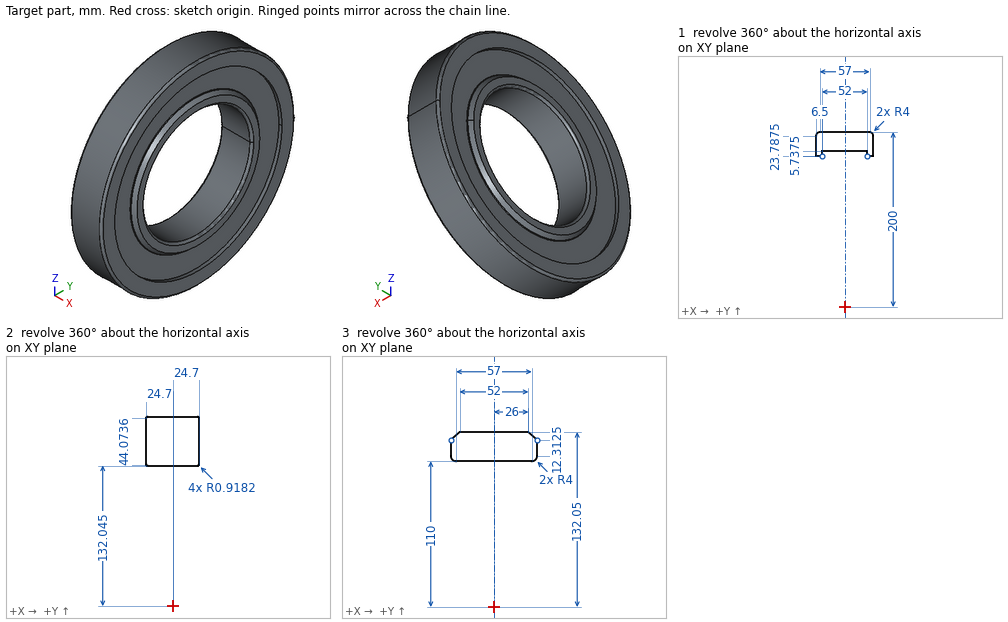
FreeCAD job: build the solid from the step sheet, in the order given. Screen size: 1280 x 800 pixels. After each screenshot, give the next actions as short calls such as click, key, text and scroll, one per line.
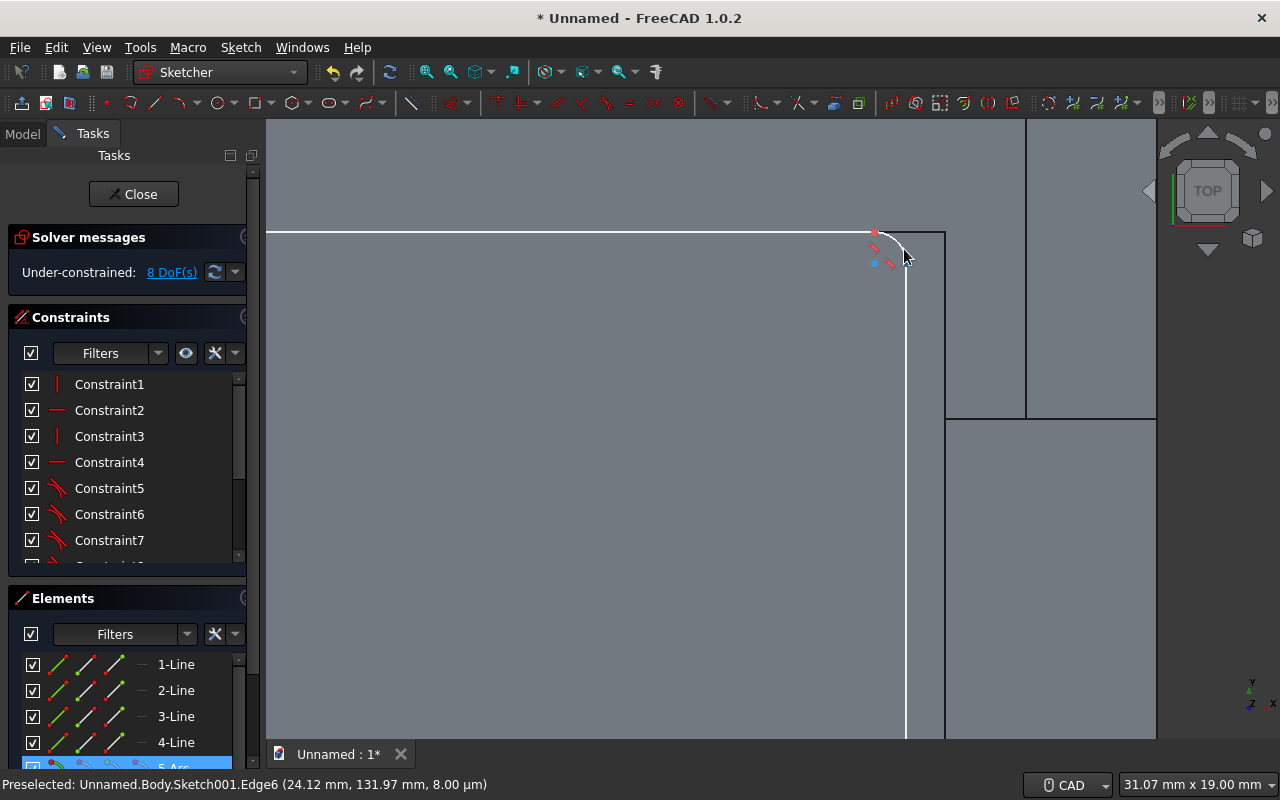
click(903, 249)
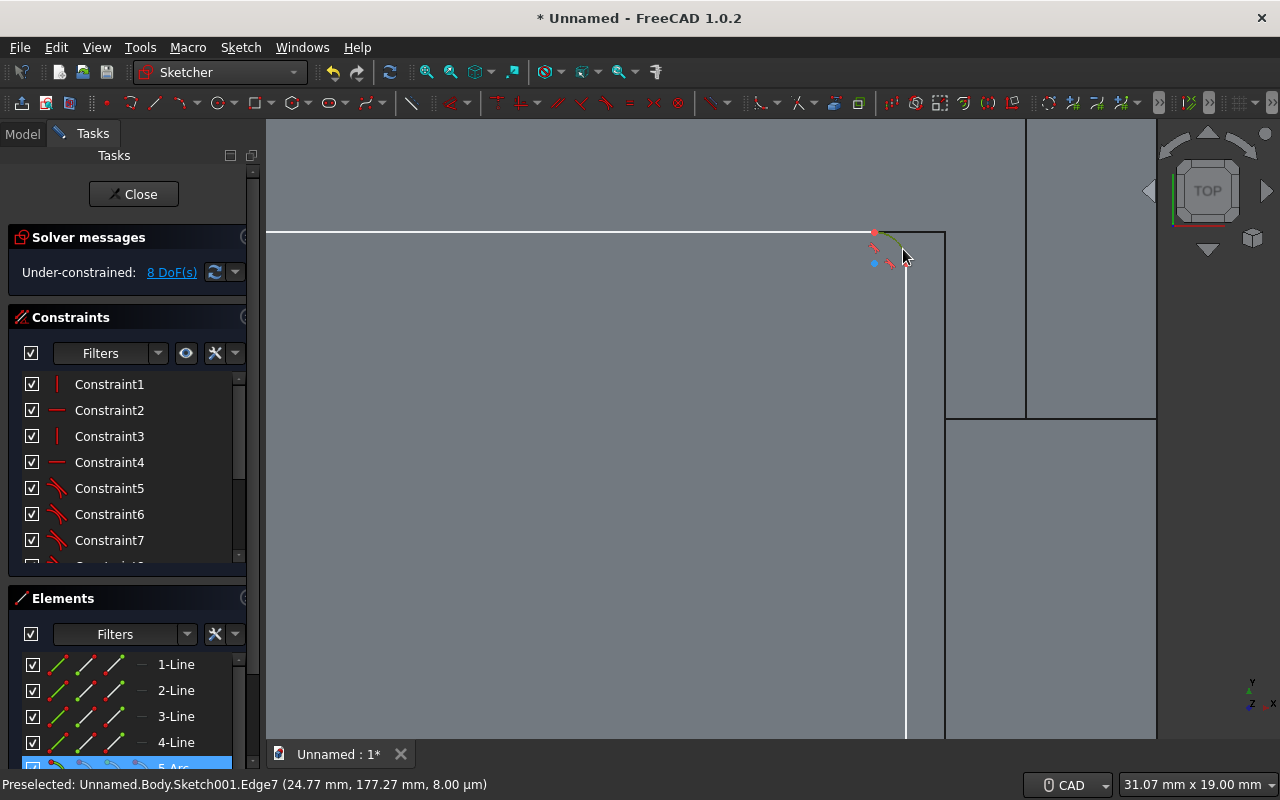
scroll(904, 248, down, 7)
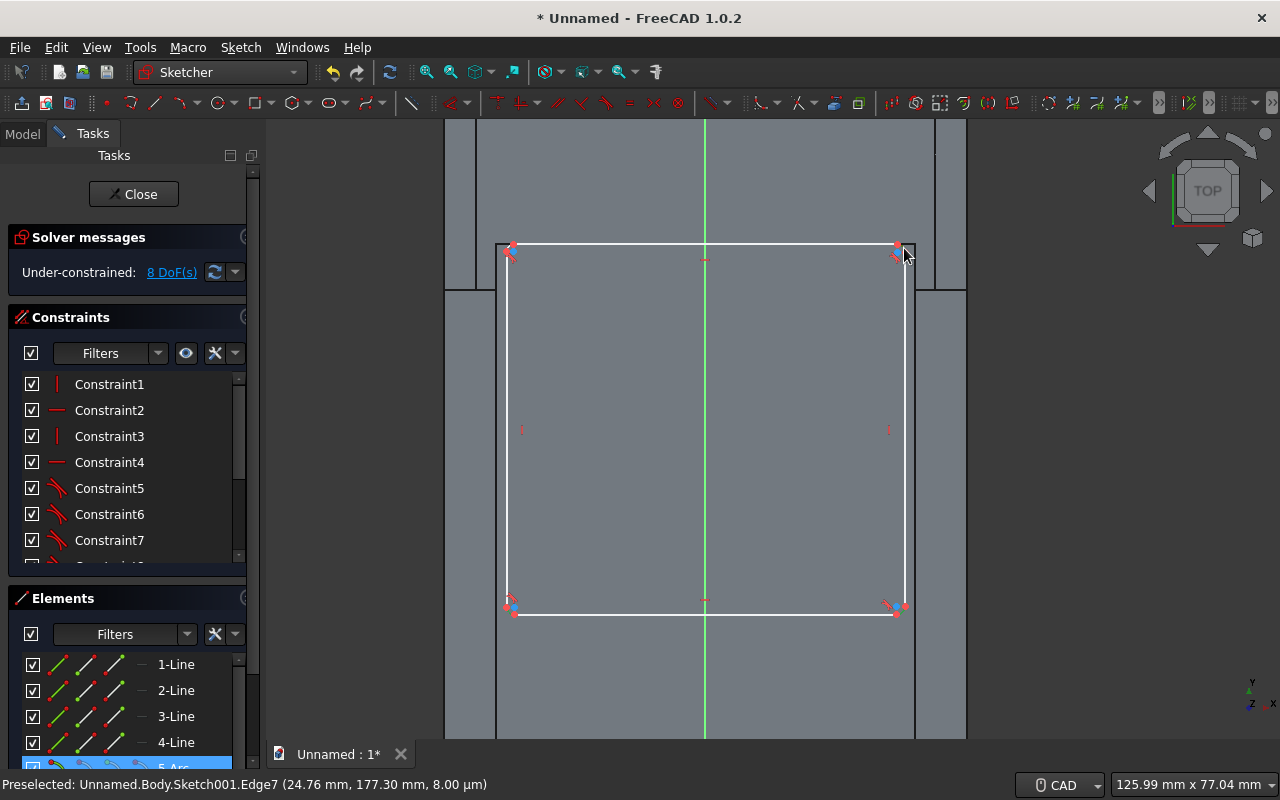
scroll(510, 245, up, 8)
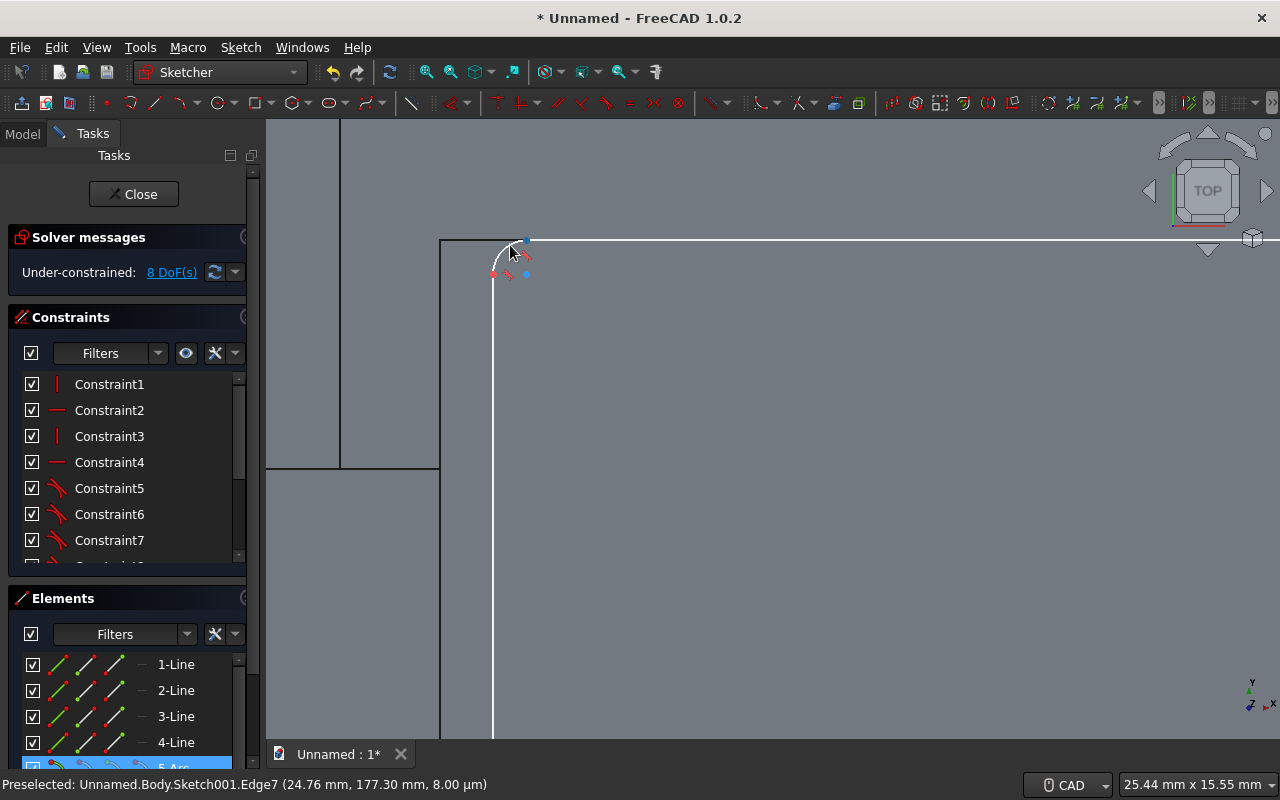
click(511, 244)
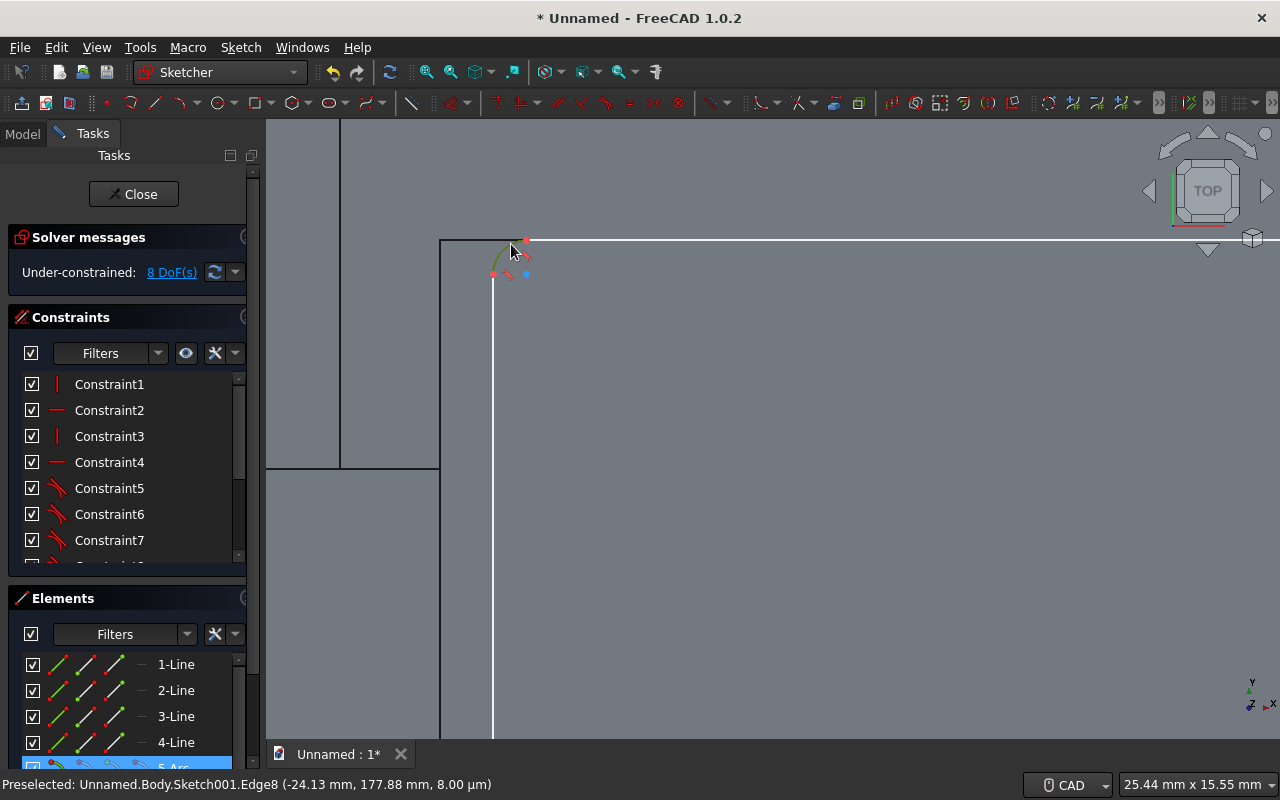
click(630, 104)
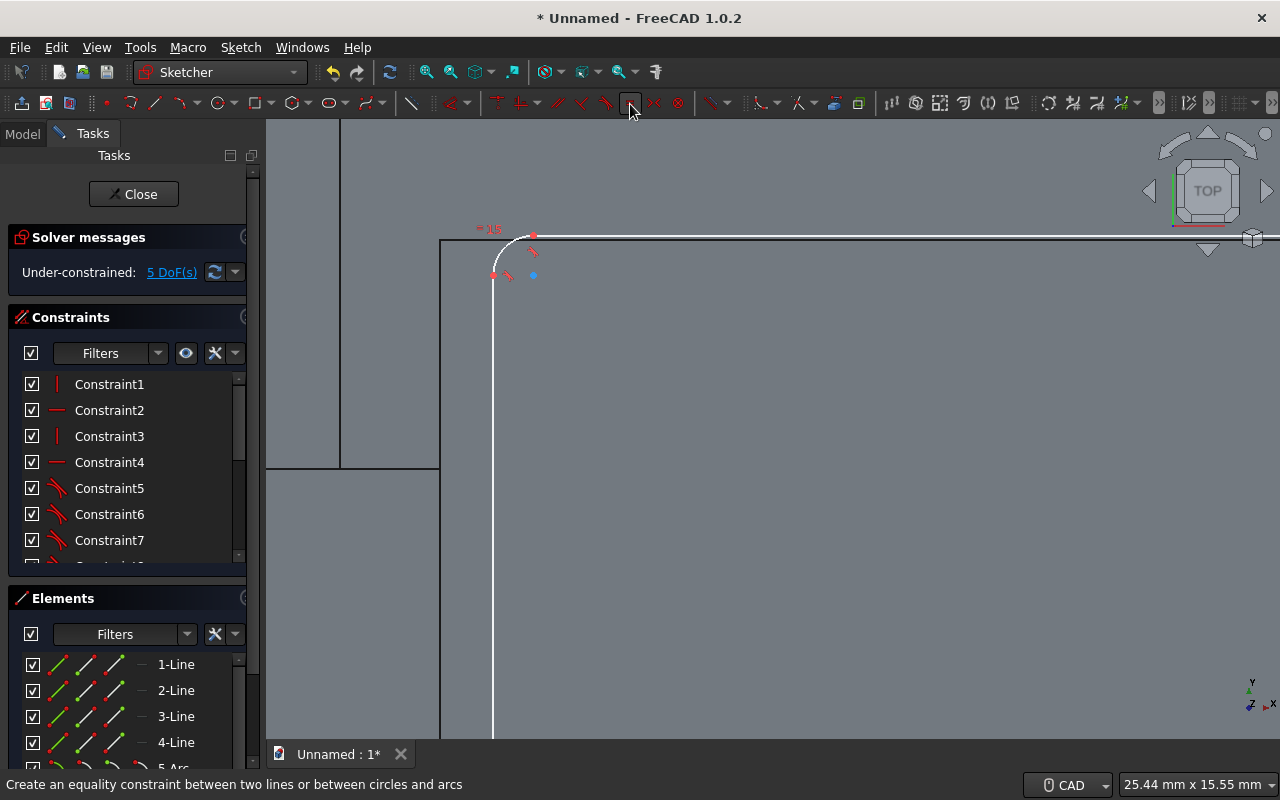
click(450, 104)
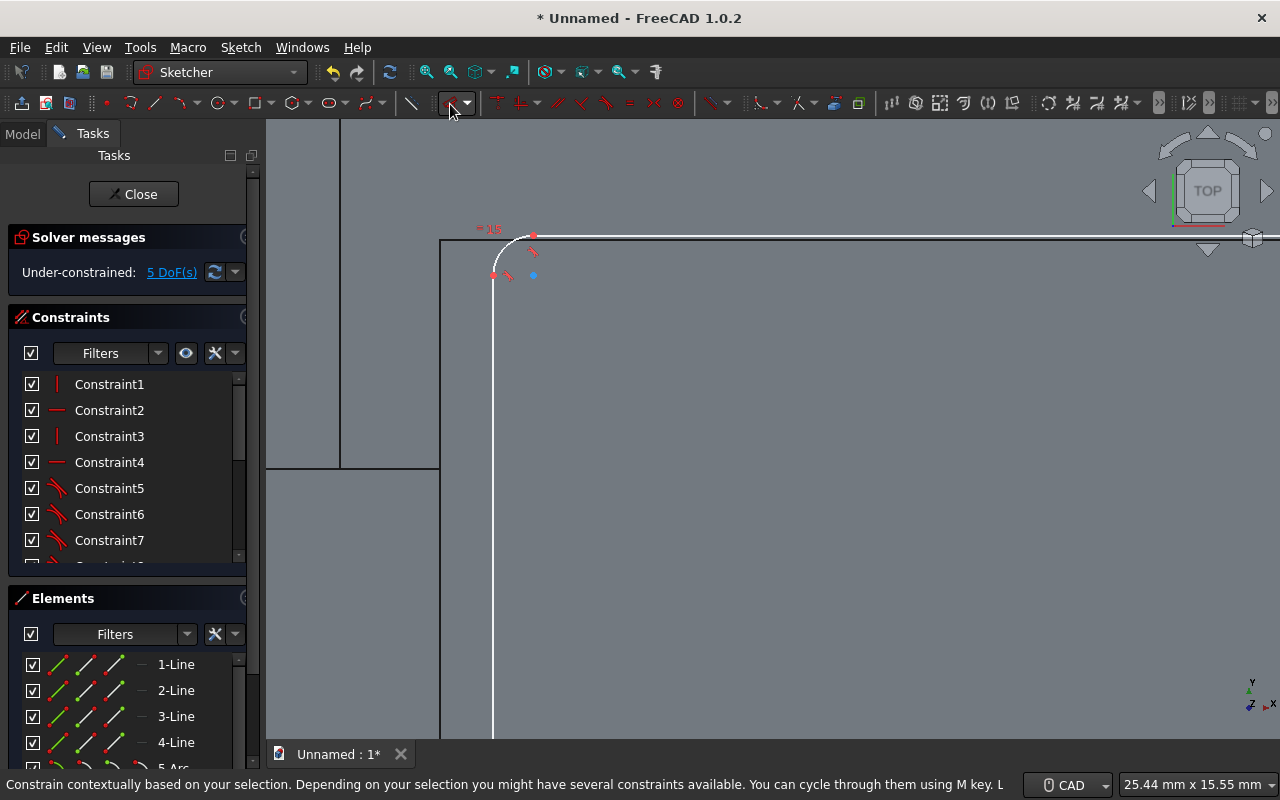
scroll(509, 245, down, 8)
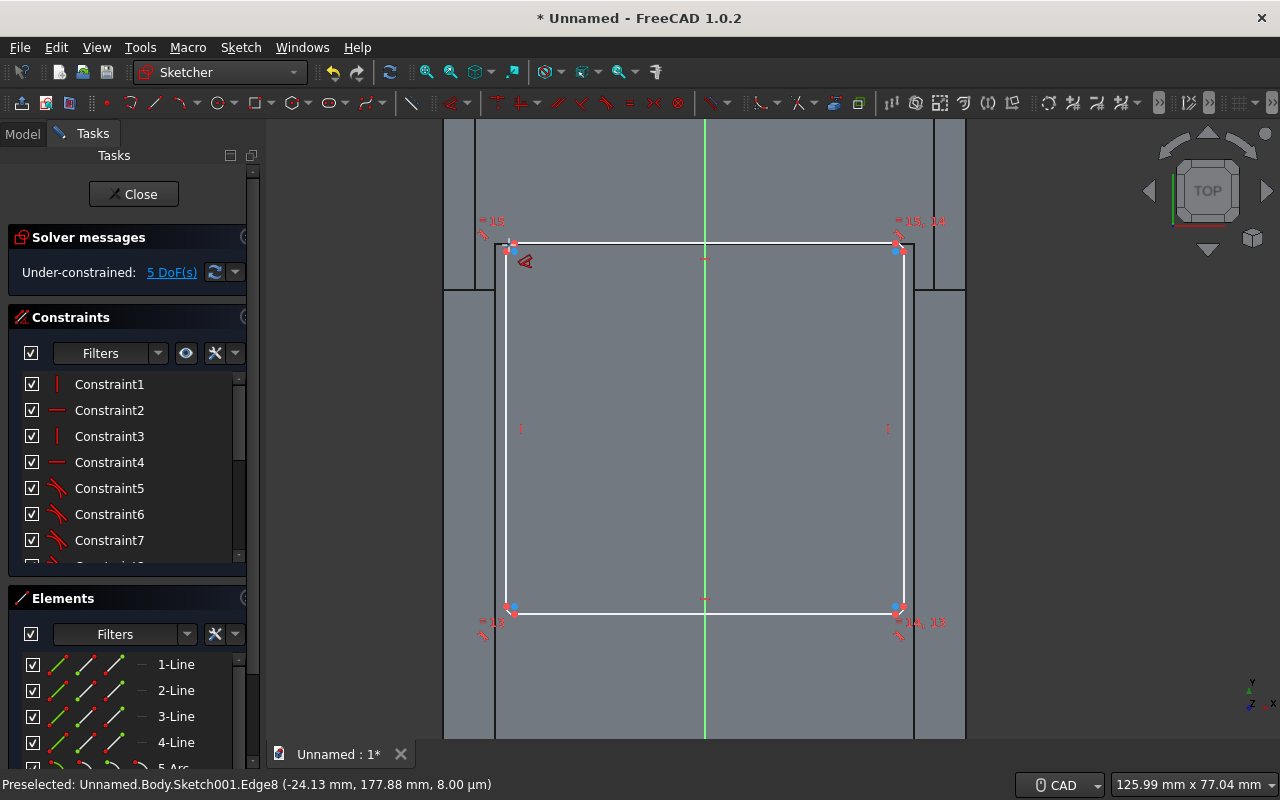
scroll(507, 610, up, 9)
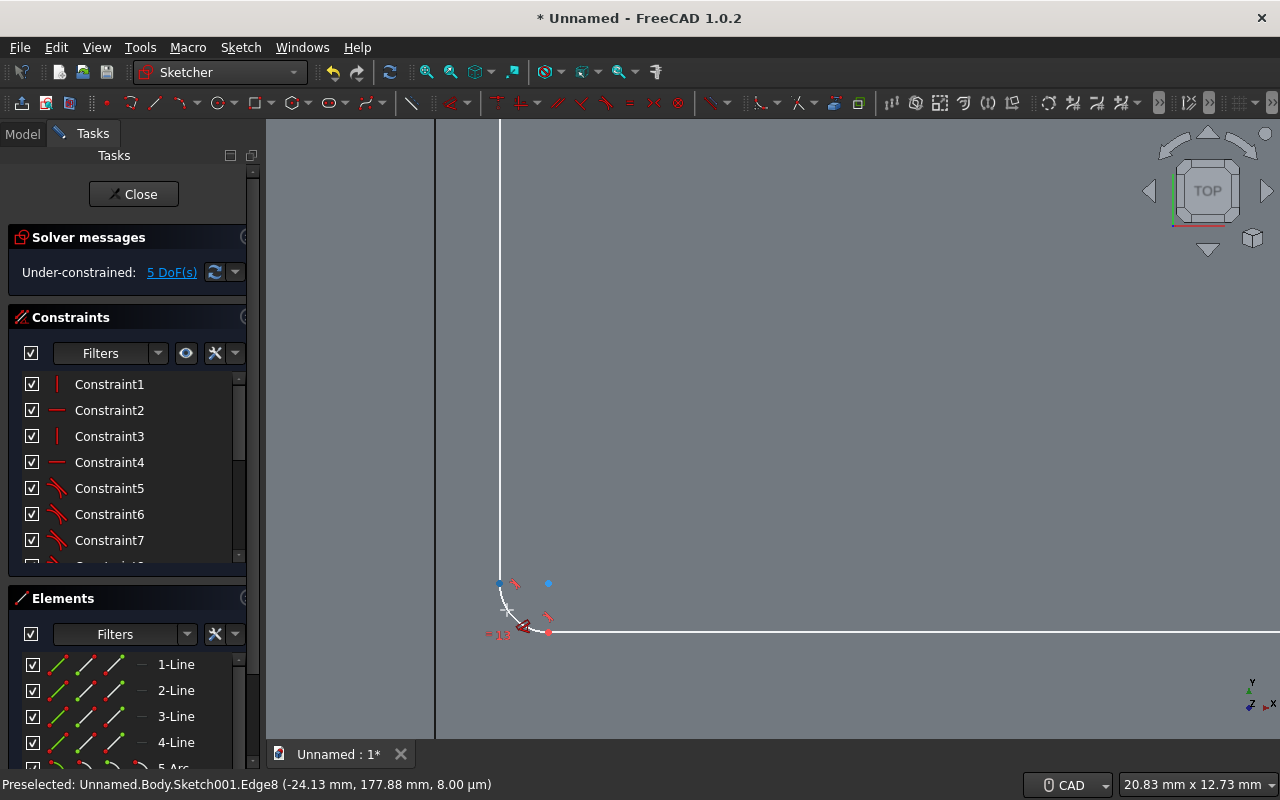
click(505, 606)
click(477, 621)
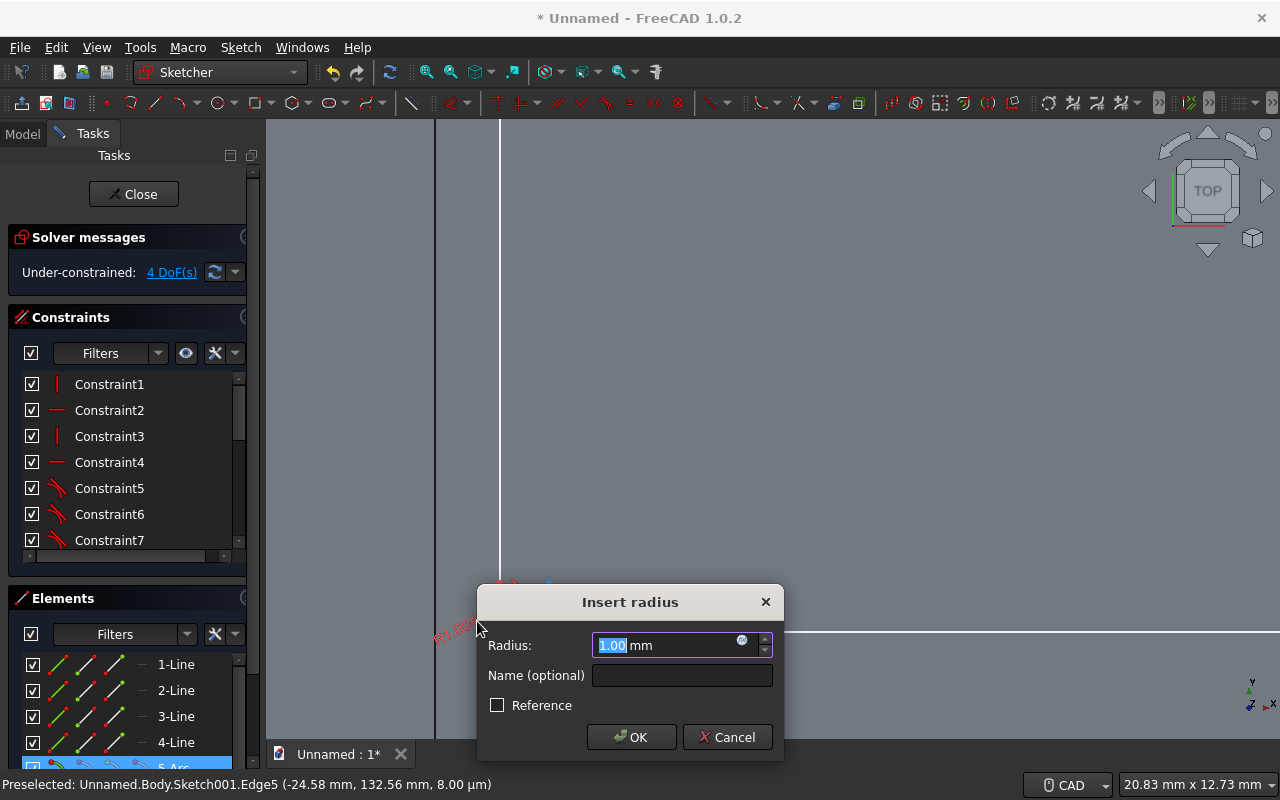
text(0.9182)
key(Return)